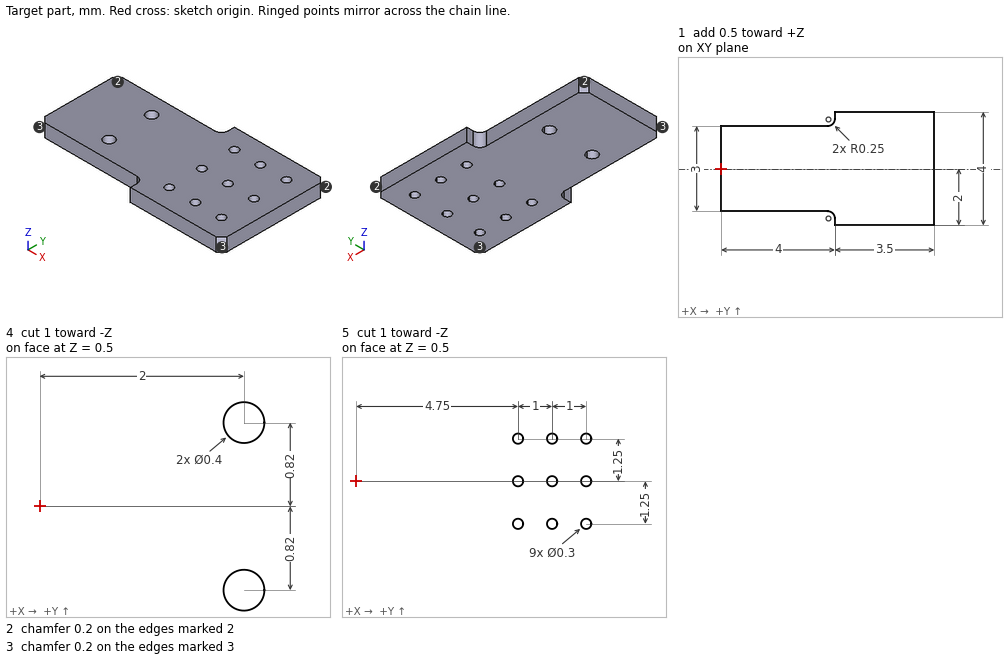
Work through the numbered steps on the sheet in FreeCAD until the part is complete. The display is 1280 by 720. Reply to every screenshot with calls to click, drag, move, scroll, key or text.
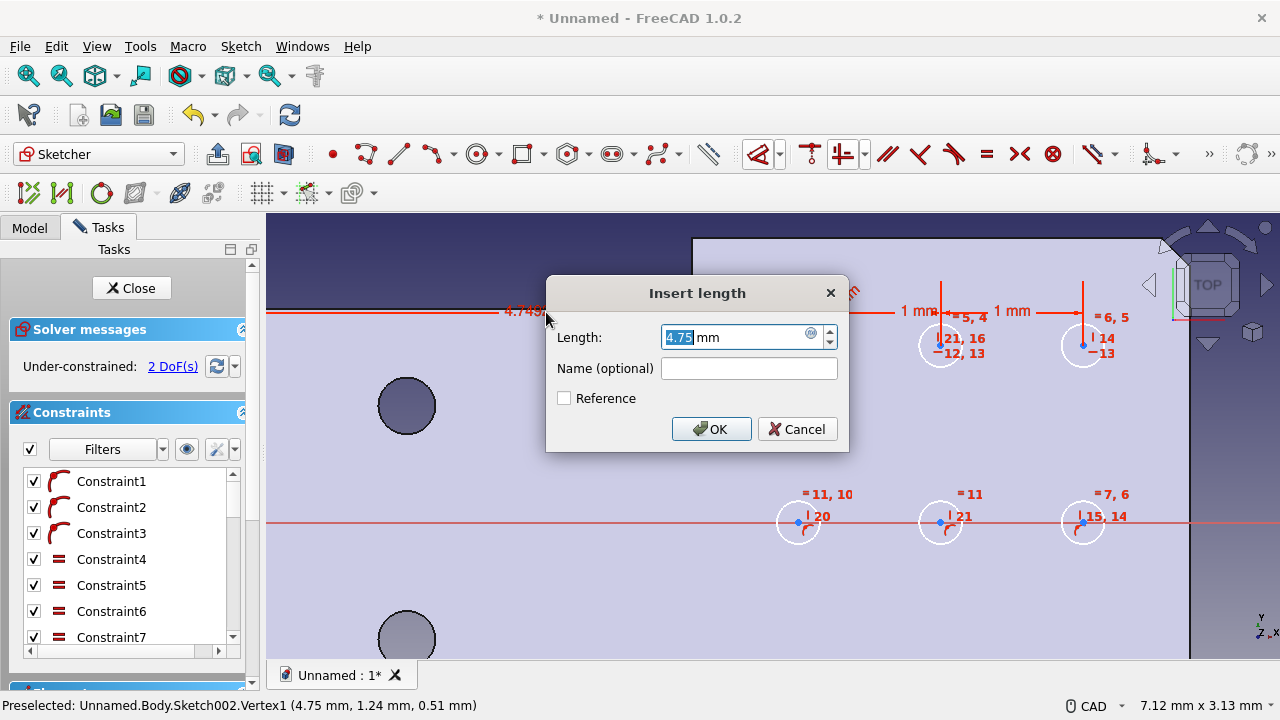
text(4.75)
key(Return)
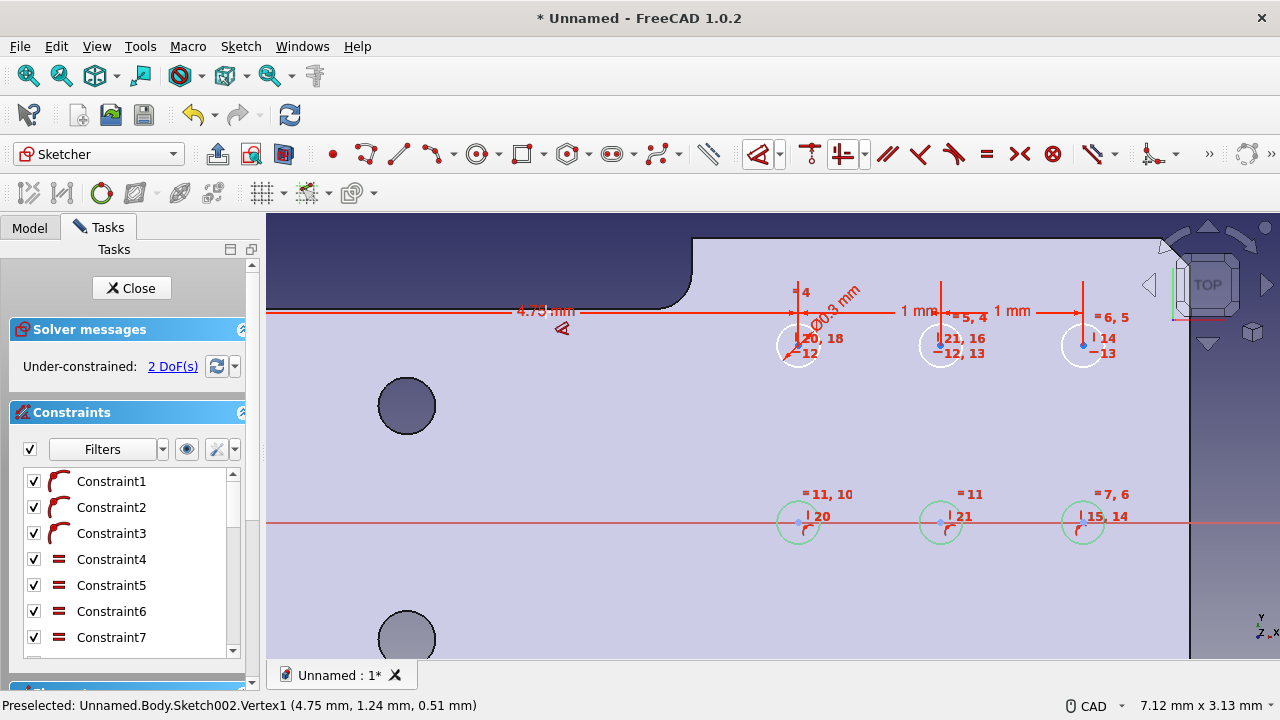
click(798, 346)
click(832, 434)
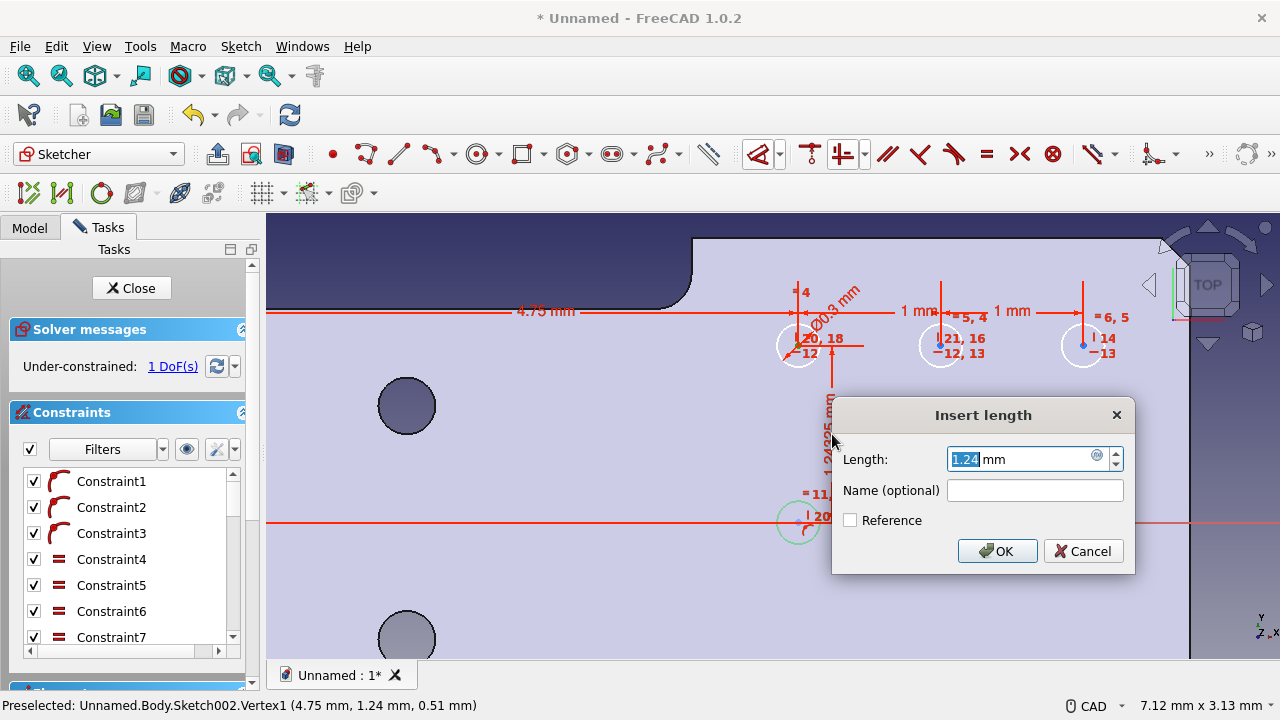
text(1.25)
key(Return)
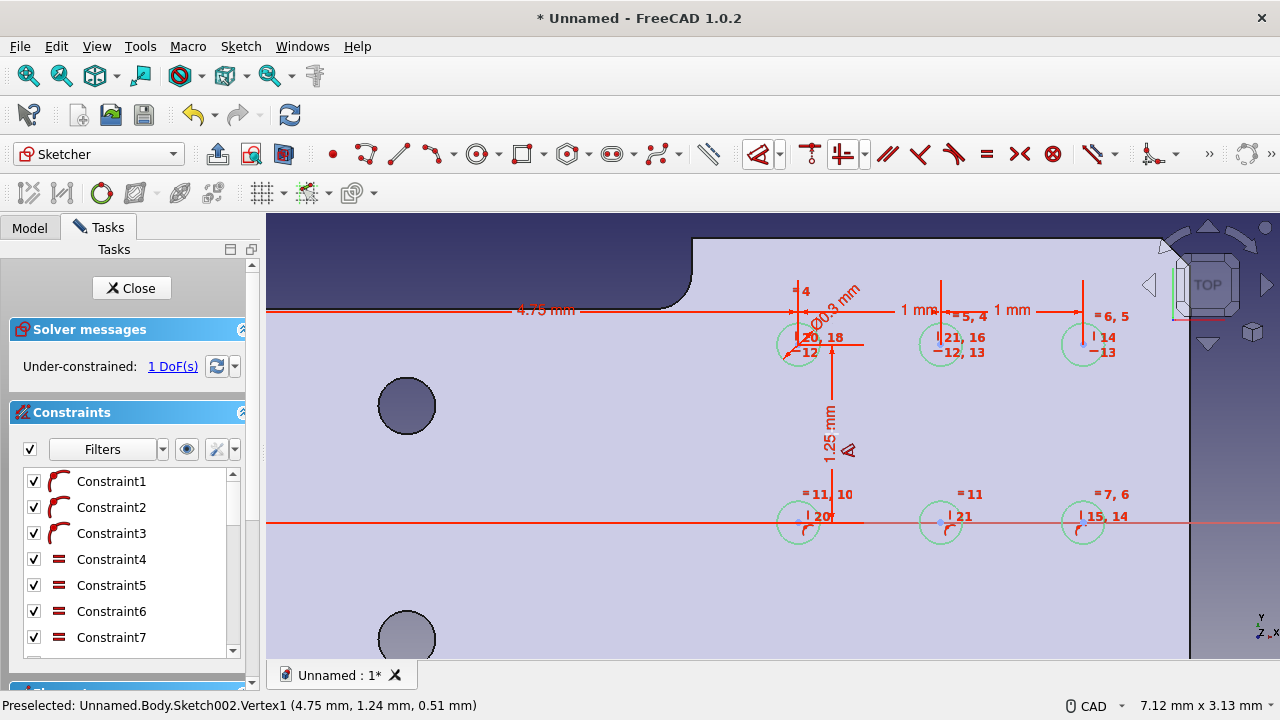
scroll(815, 331, down, 3)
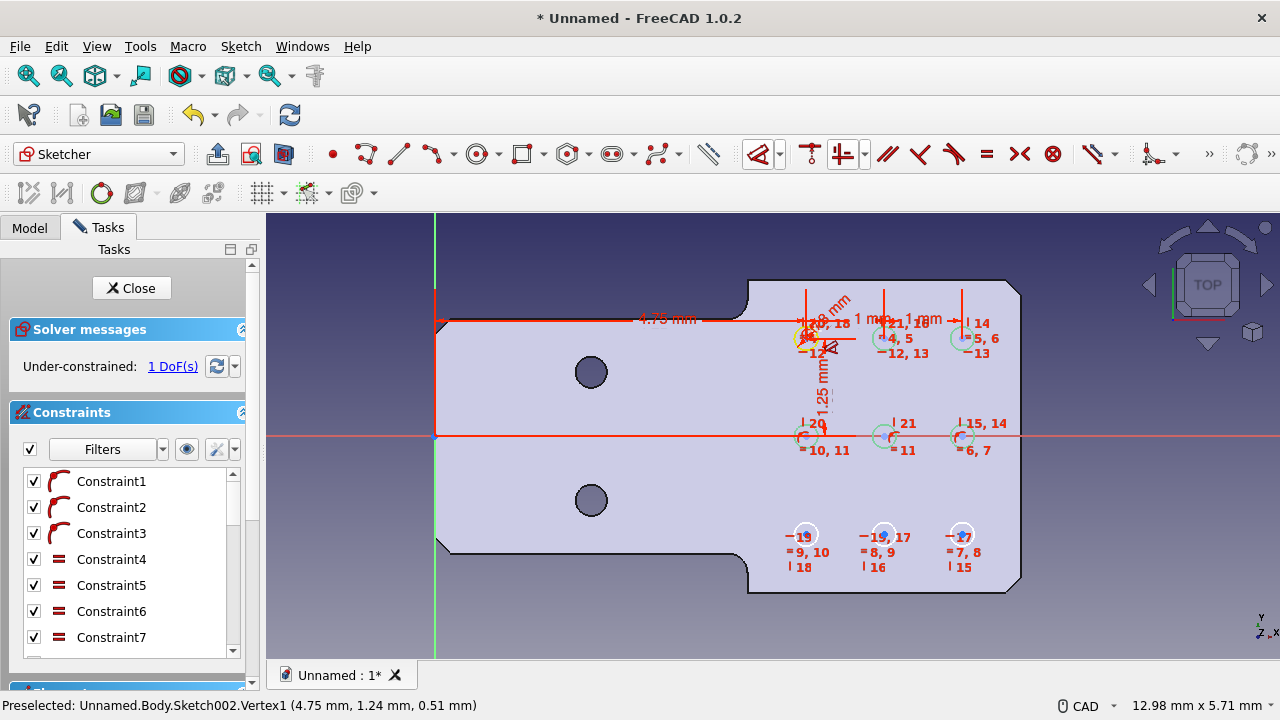
click(962, 534)
click(401, 485)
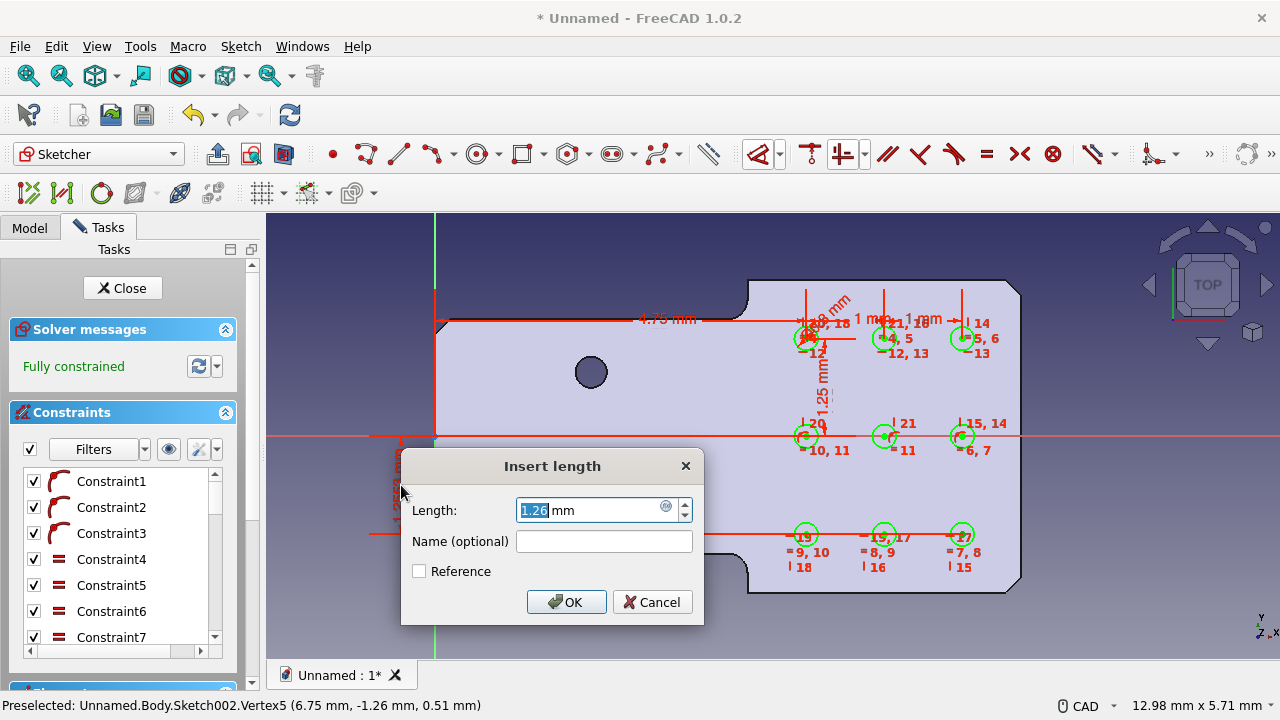
text(1.25)
key(Return)
key(Escape)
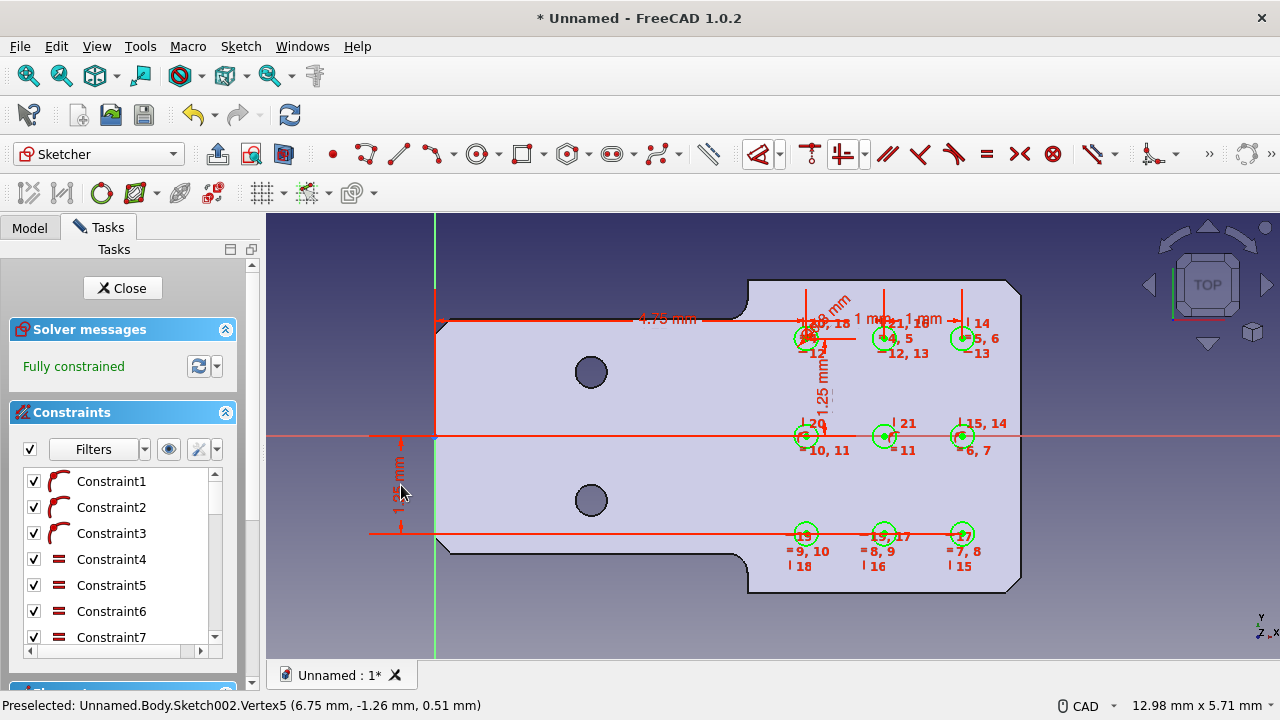
click(123, 288)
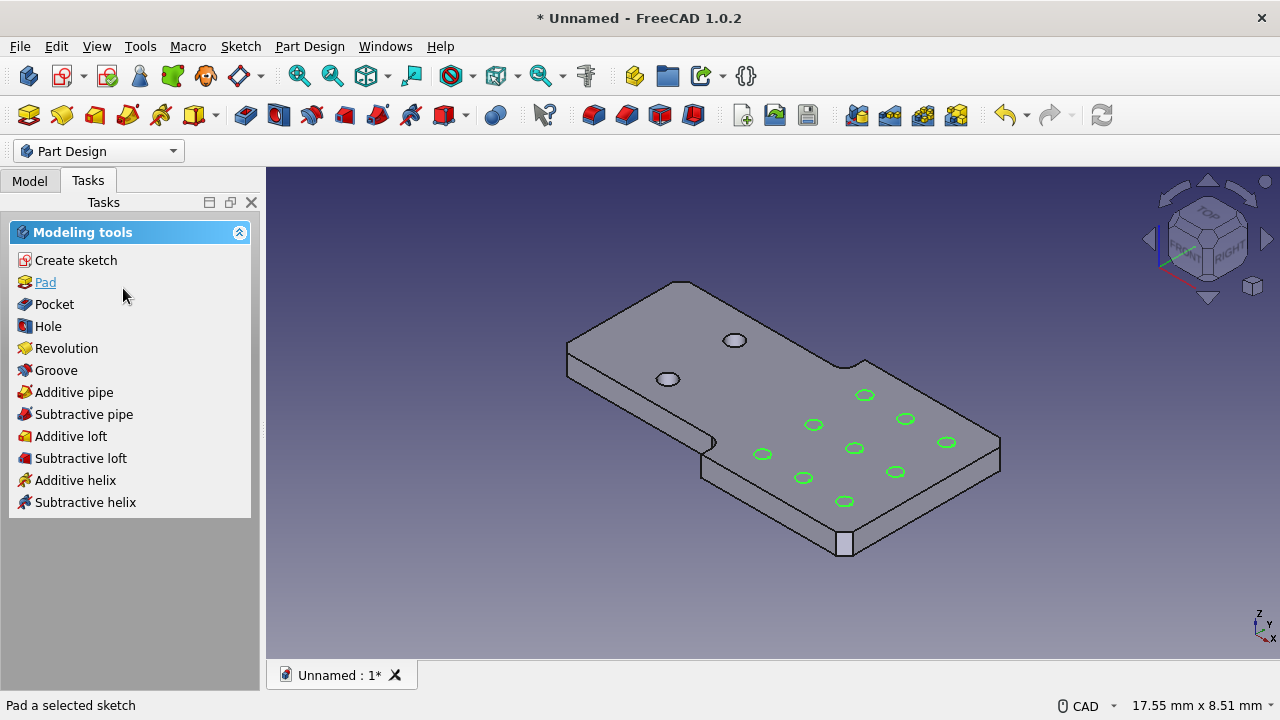
click(246, 116)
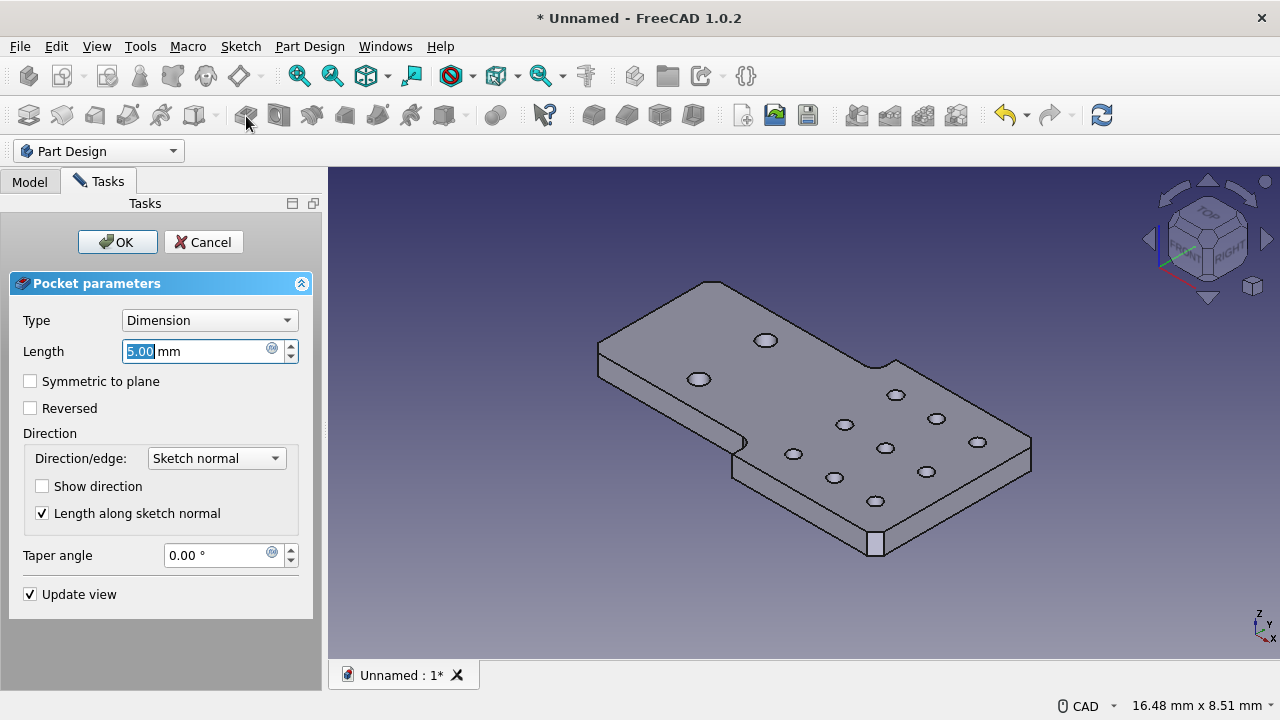
text(1)
key(Tab)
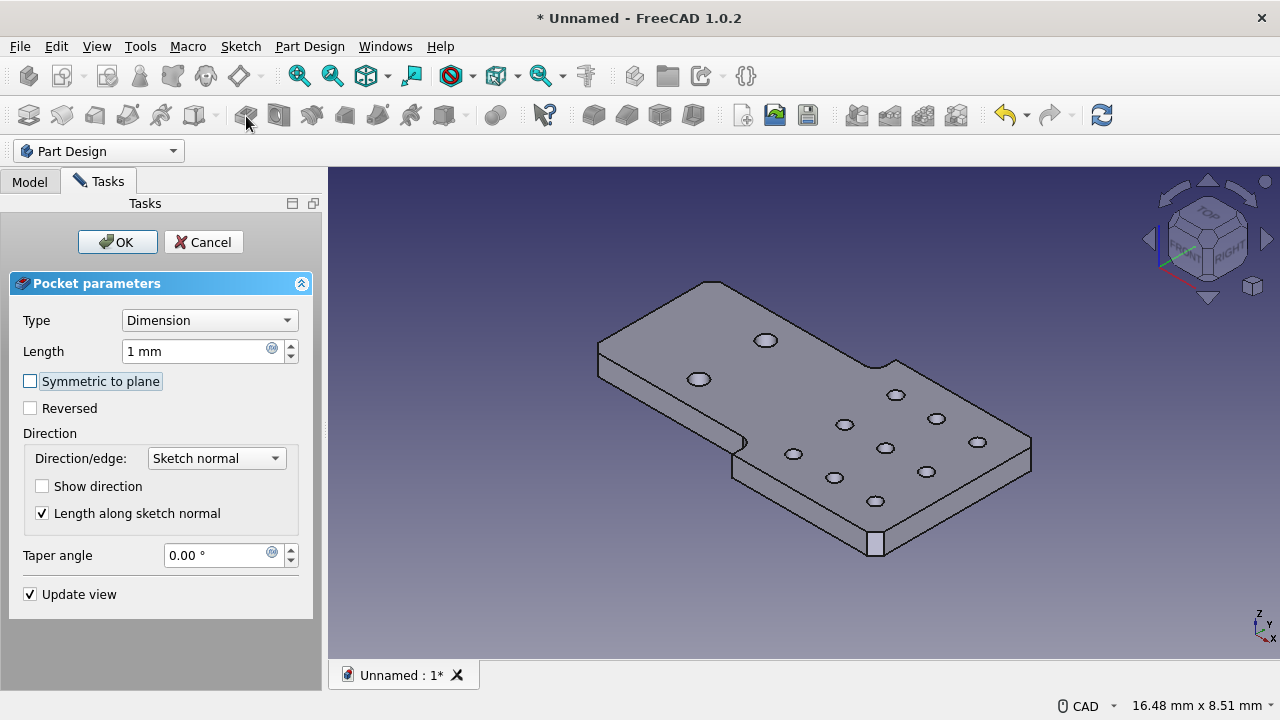
click(118, 242)